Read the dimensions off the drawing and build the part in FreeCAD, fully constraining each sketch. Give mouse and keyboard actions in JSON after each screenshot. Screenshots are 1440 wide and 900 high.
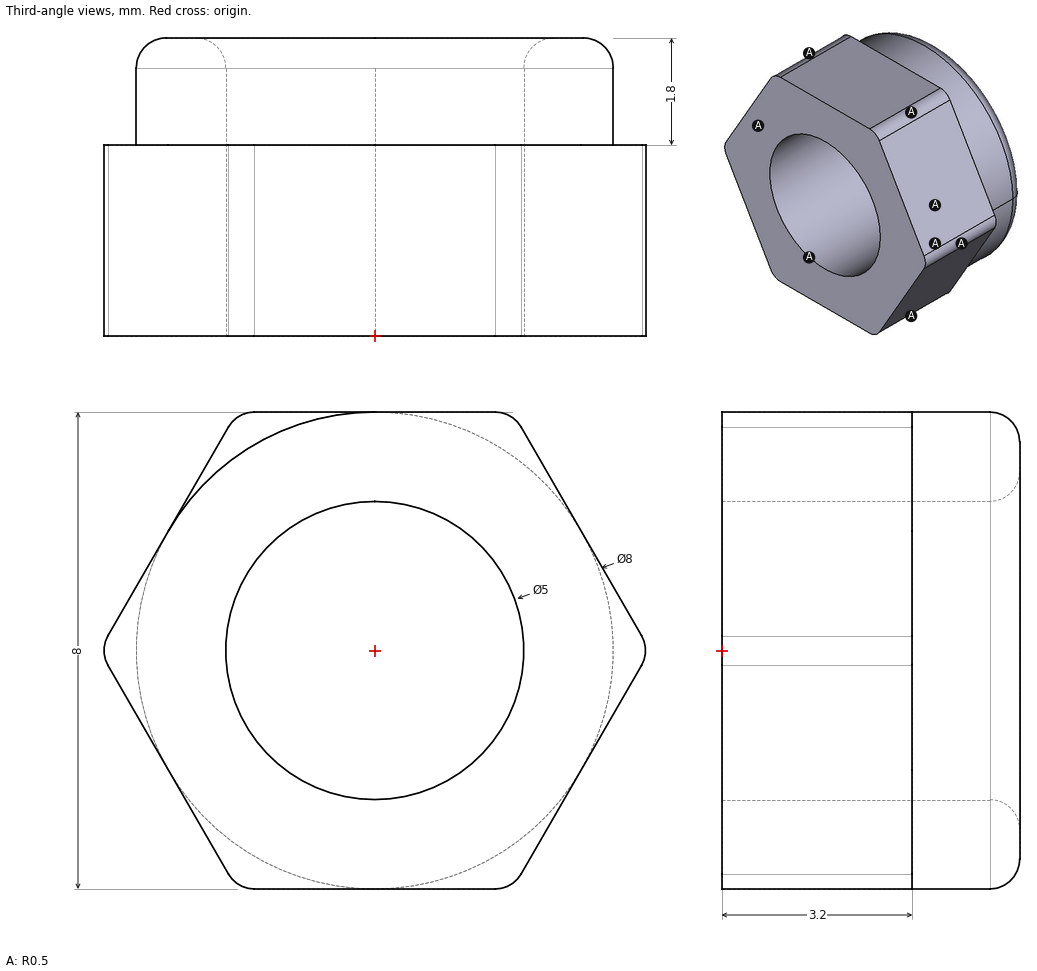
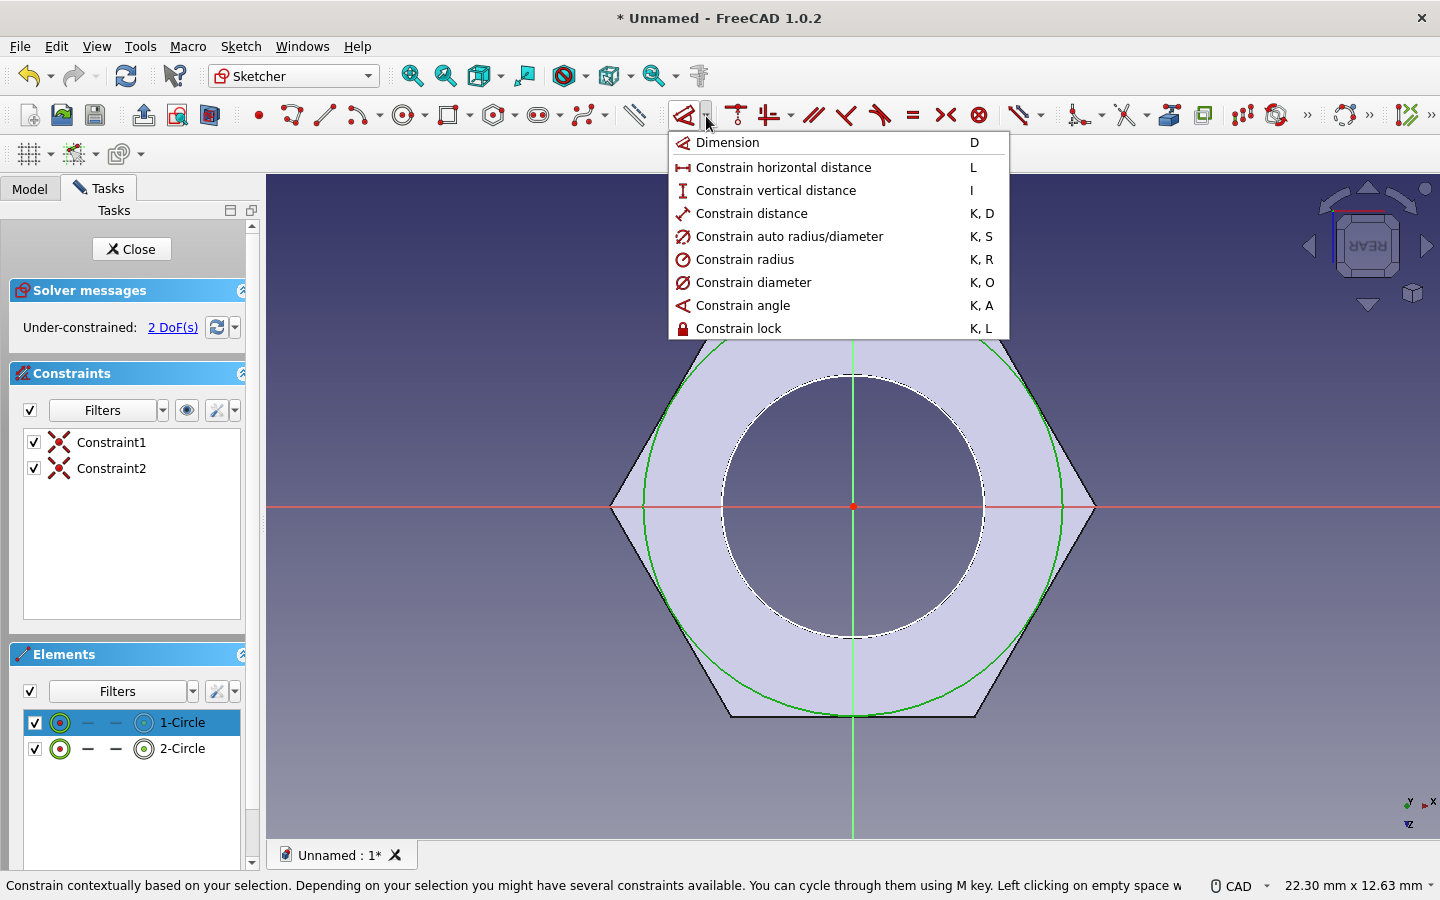
{"action": "left_click", "coordinate": [839, 282]}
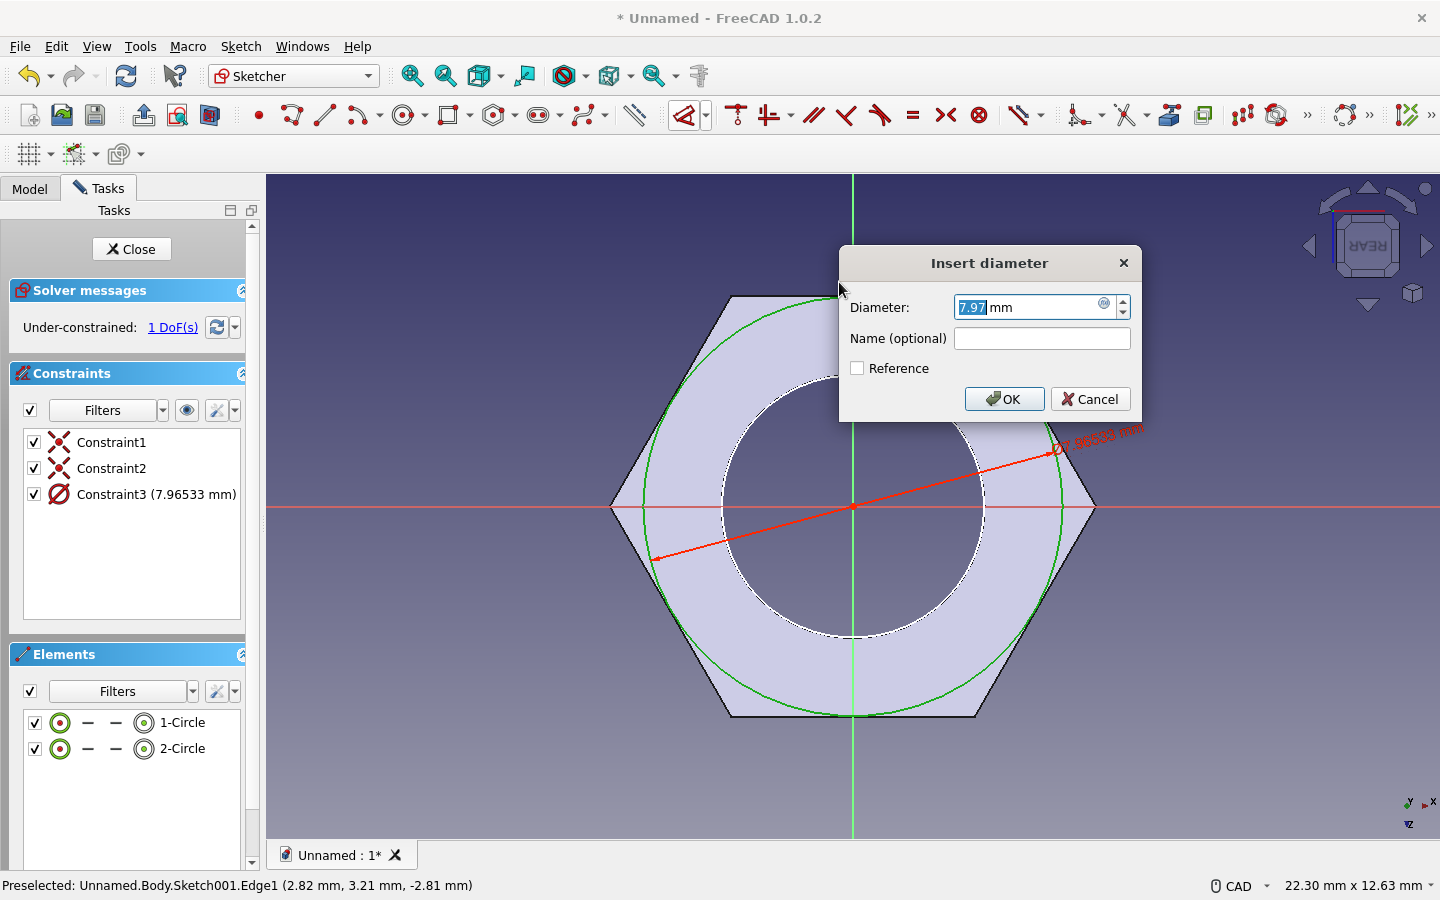
{"action": "type", "text": "8"}
{"action": "key", "text": "Return"}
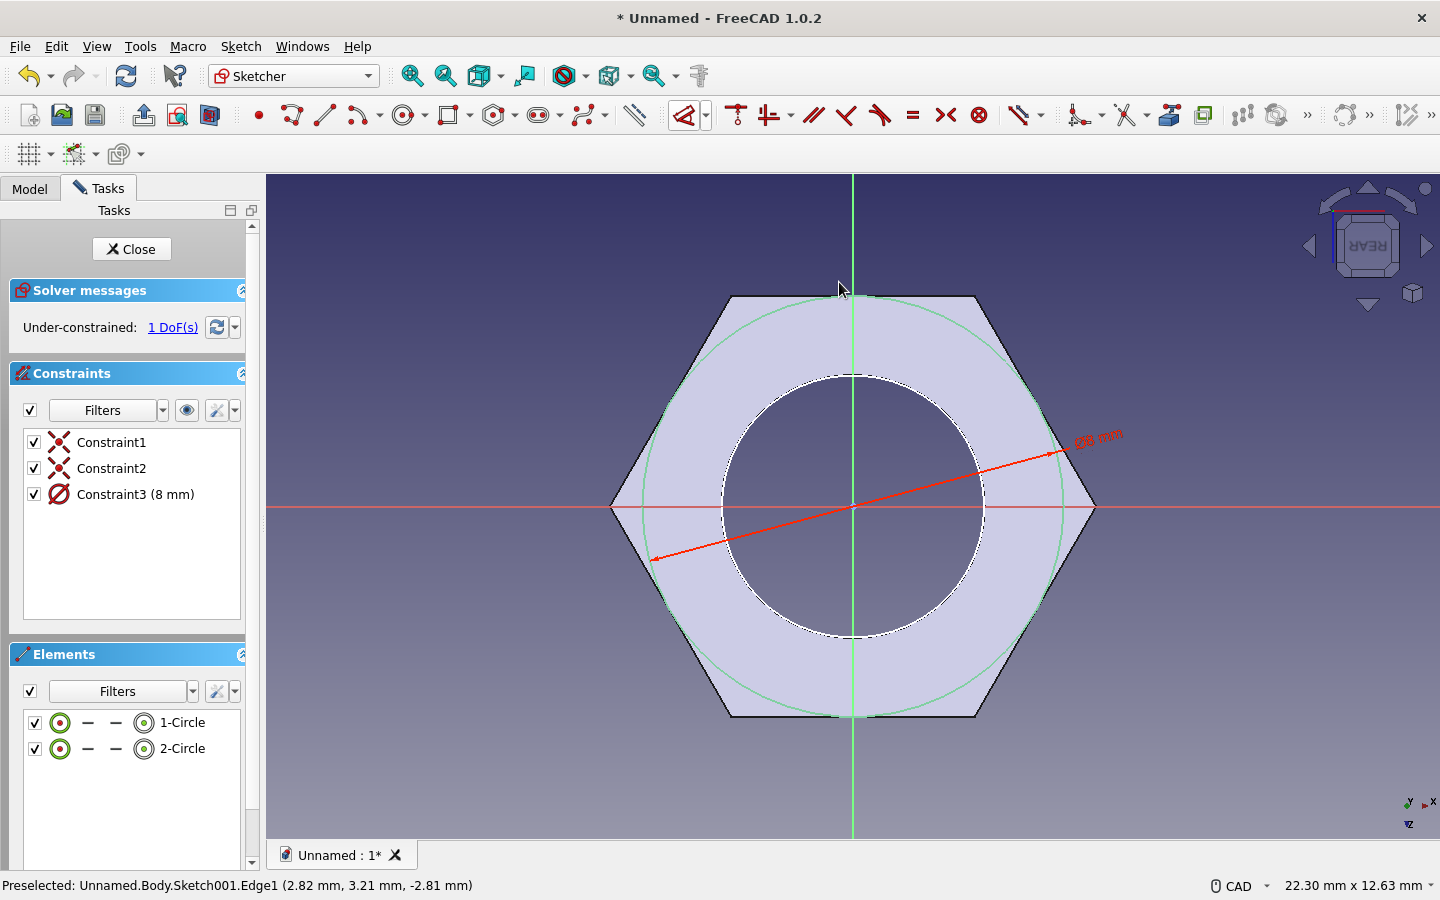
{"action": "left_click", "coordinate": [945, 413]}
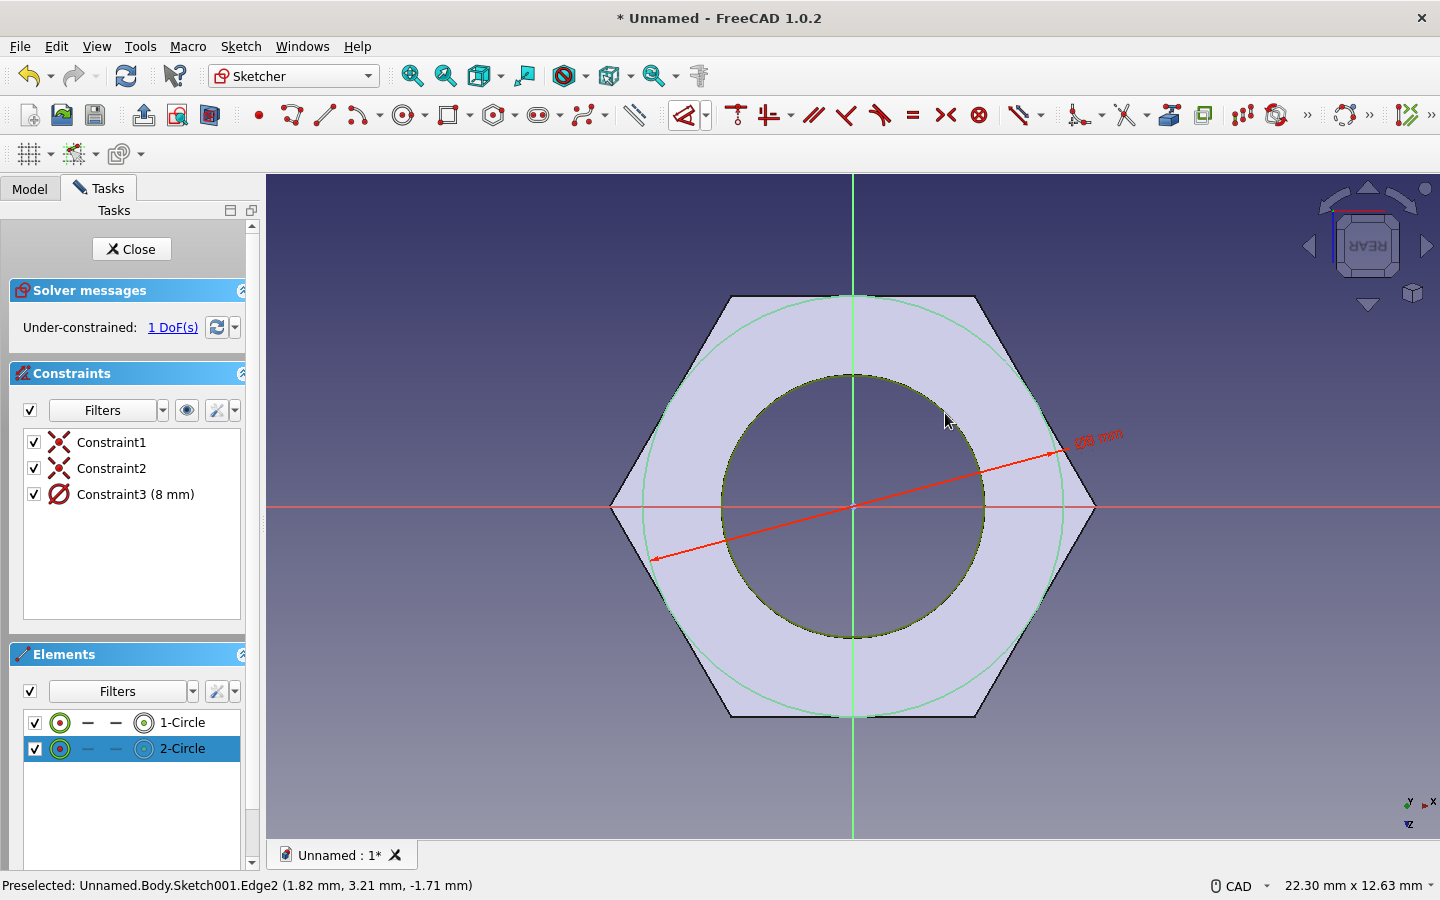
{"action": "left_click", "coordinate": [706, 116]}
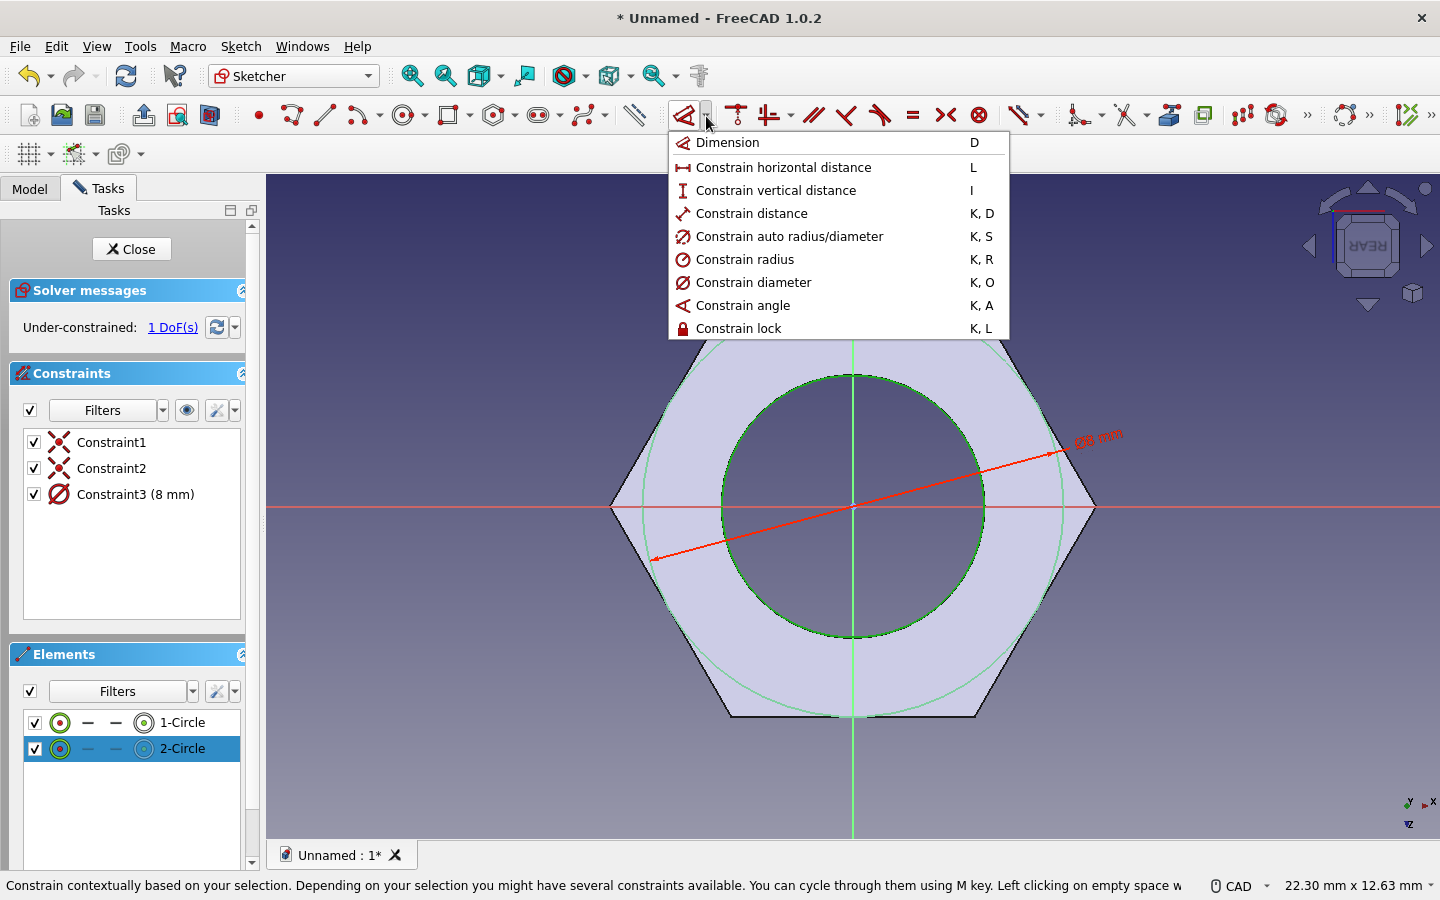
{"action": "left_click", "coordinate": [839, 282]}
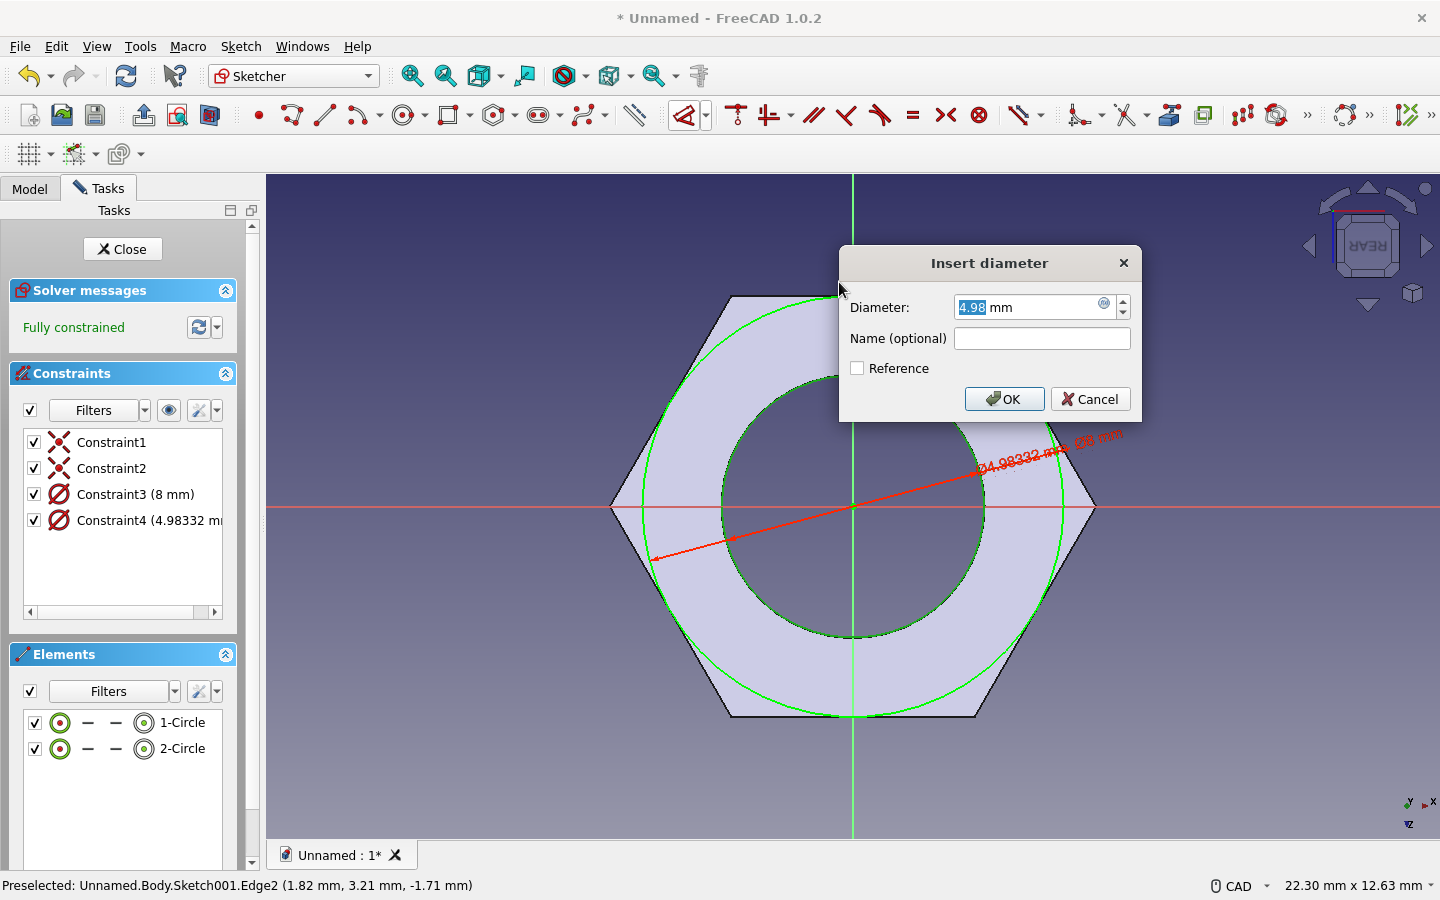
{"action": "type", "text": "5"}
{"action": "key", "text": "Return"}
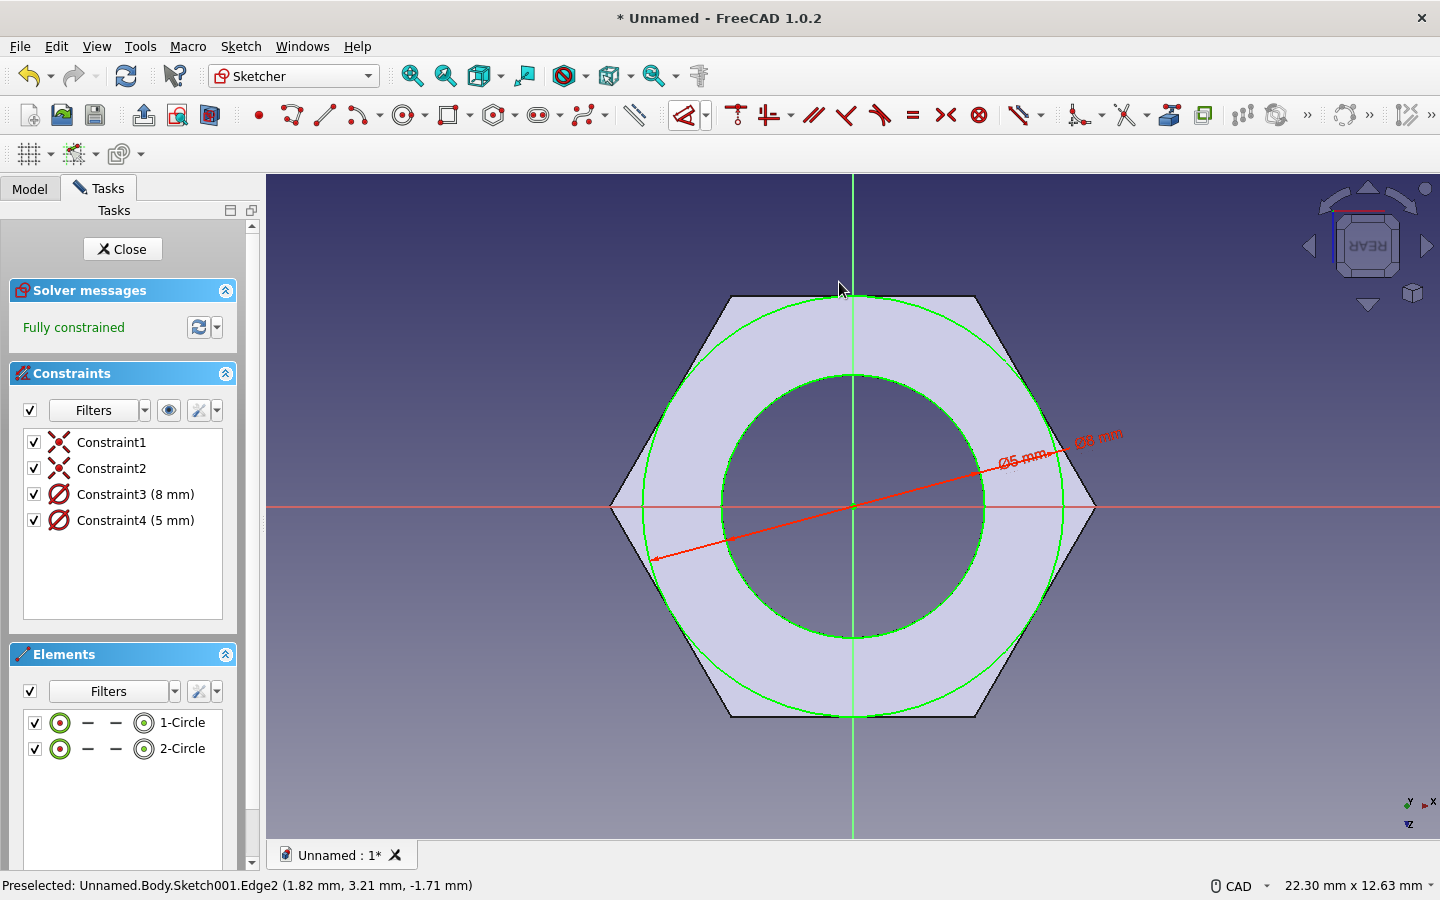
{"action": "left_click", "coordinate": [123, 249]}